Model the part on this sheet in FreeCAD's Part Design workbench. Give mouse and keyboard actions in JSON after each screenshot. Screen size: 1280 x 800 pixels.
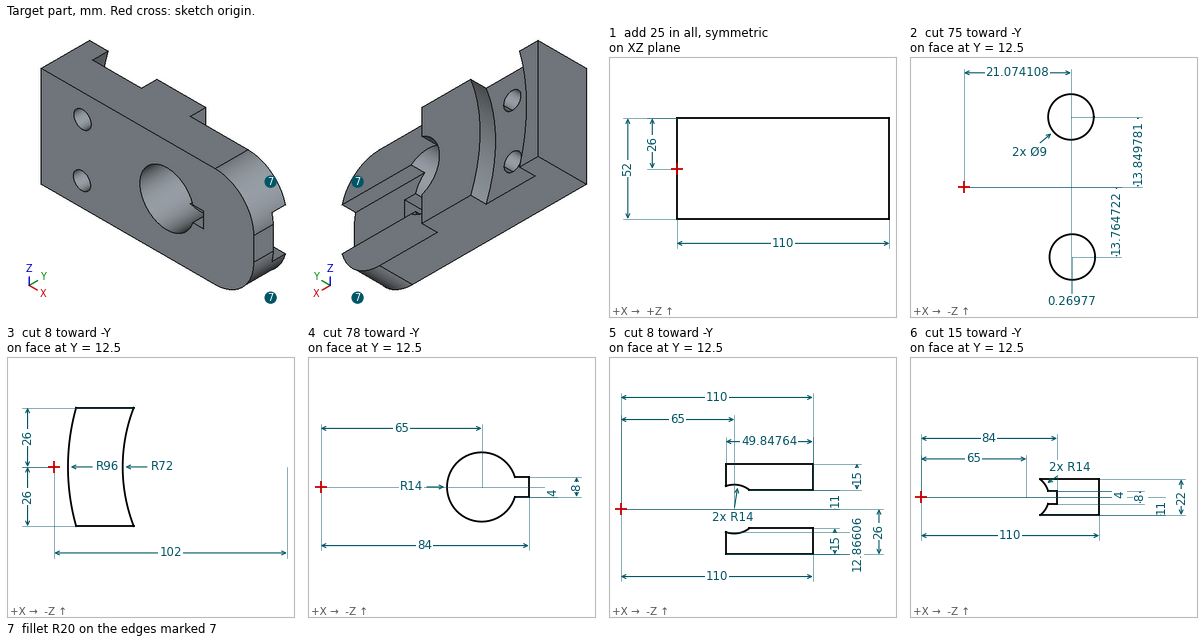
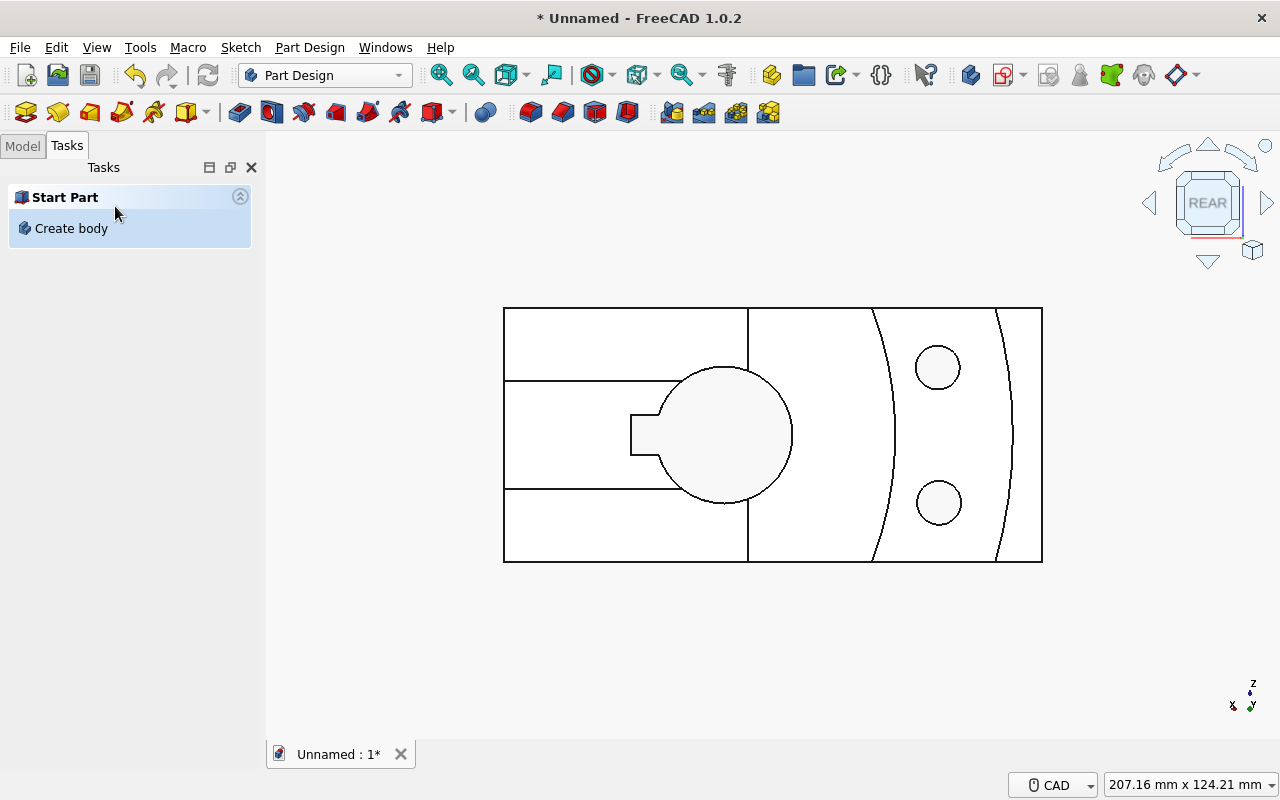
{"action": "left_click", "coordinate": [822, 507]}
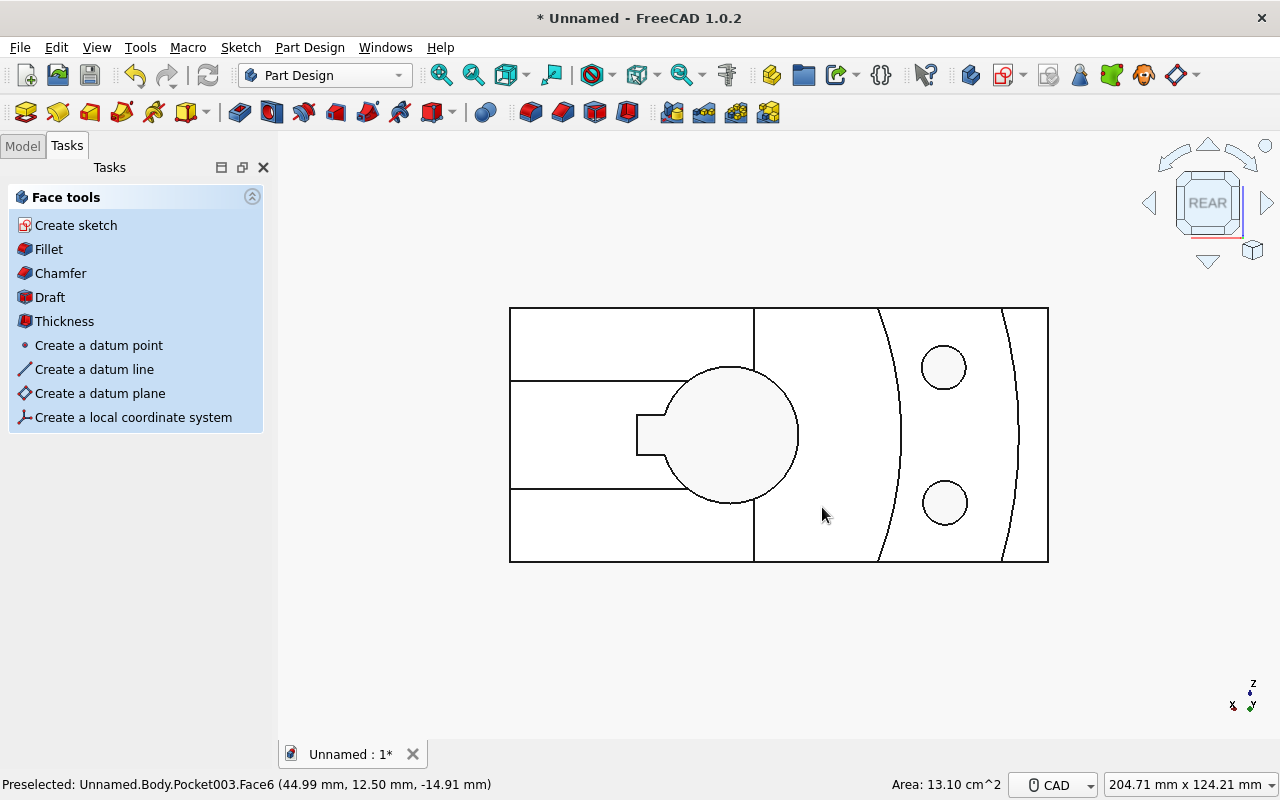
{"action": "left_click", "coordinate": [1004, 76]}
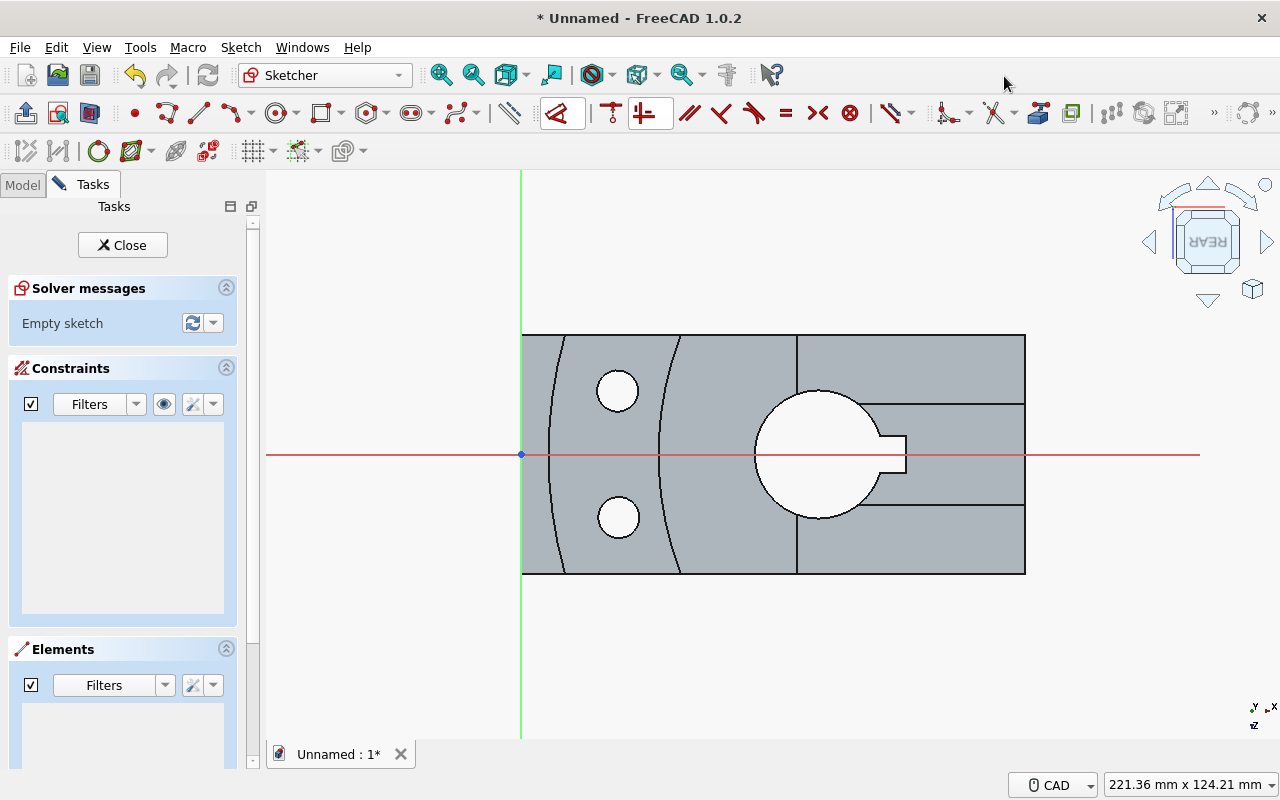
{"action": "scroll", "coordinate": [1044, 454], "scroll_direction": "up", "scroll_amount": 6}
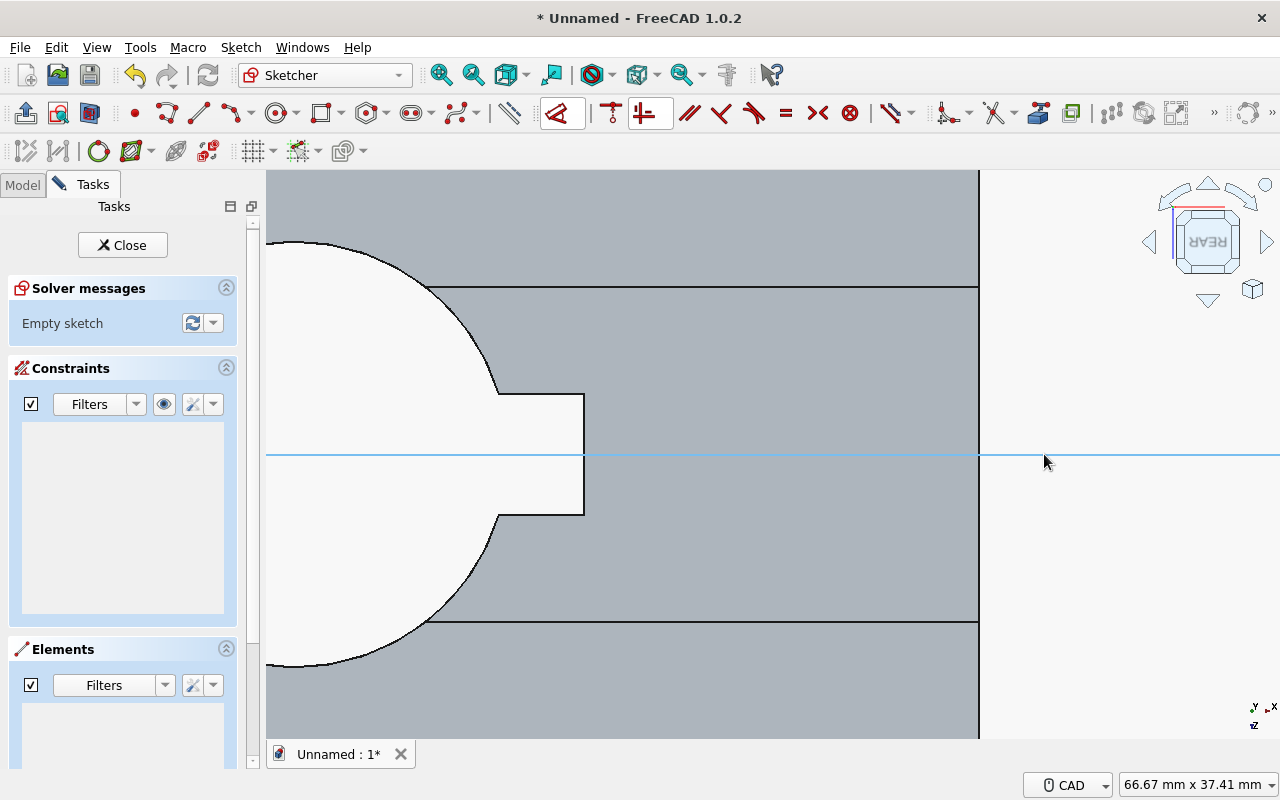
{"action": "left_click", "coordinate": [168, 114]}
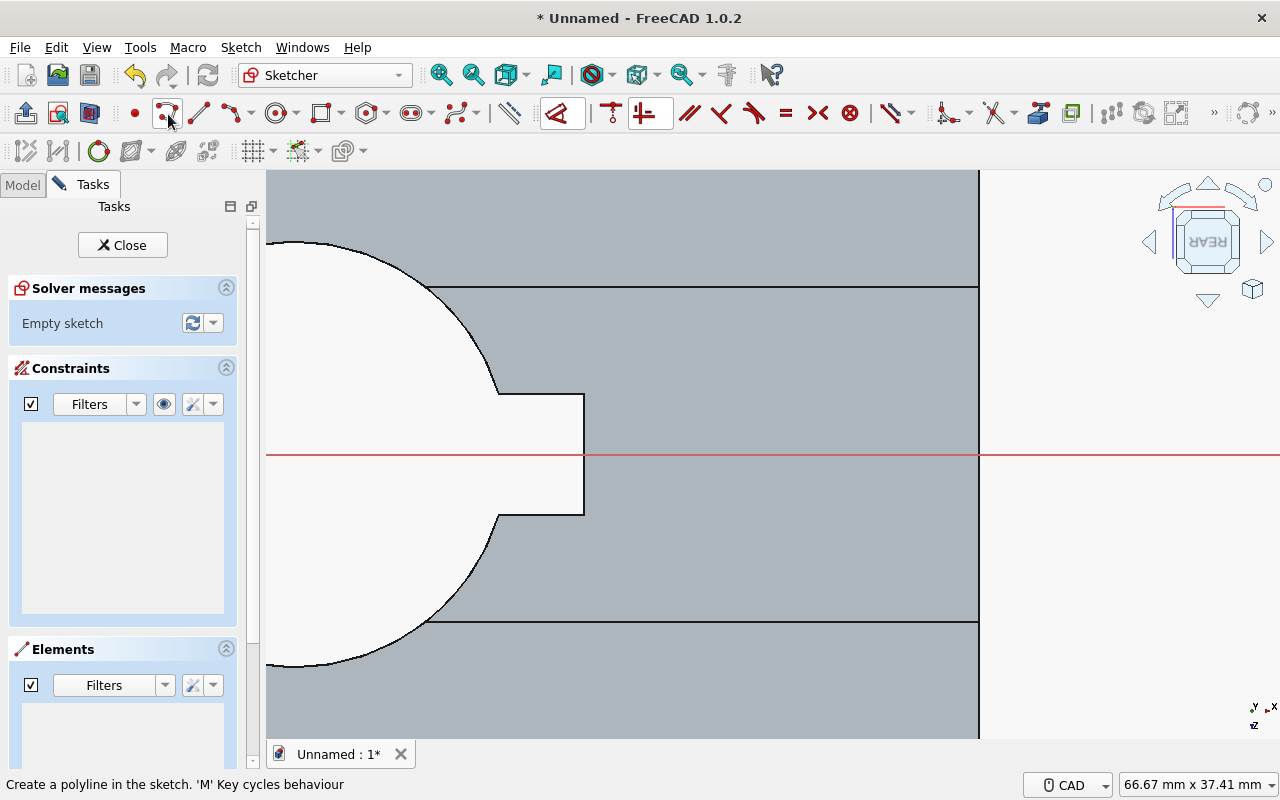
{"action": "left_click", "coordinate": [499, 394]}
{"action": "left_click", "coordinate": [584, 394]}
{"action": "left_click", "coordinate": [584, 515]}
{"action": "left_click", "coordinate": [499, 515]}
{"action": "right_click", "coordinate": [499, 515]}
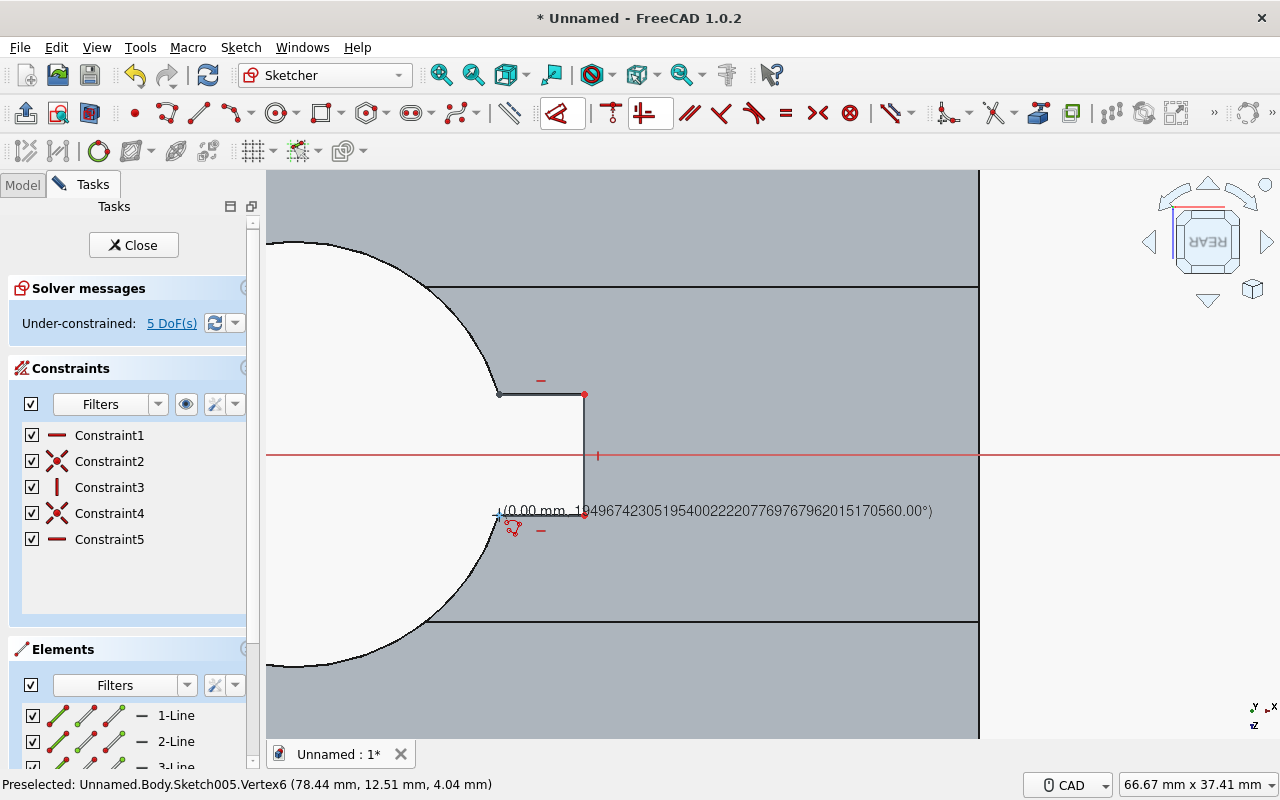
{"action": "left_click", "coordinate": [426, 622]}
{"action": "left_click", "coordinate": [979, 622]}
{"action": "left_click", "coordinate": [979, 287]}
{"action": "left_click", "coordinate": [426, 287]}
{"action": "right_click", "coordinate": [426, 287]}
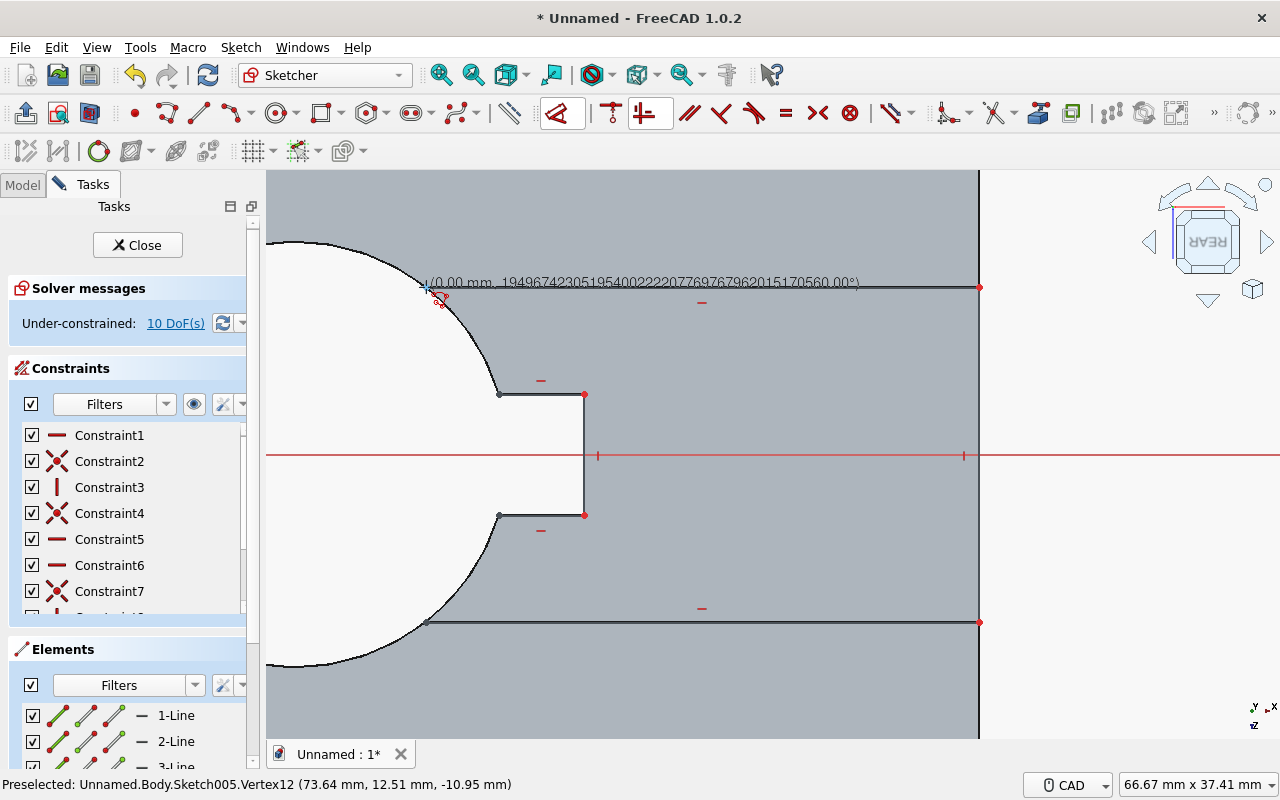
{"action": "left_click", "coordinate": [232, 114]}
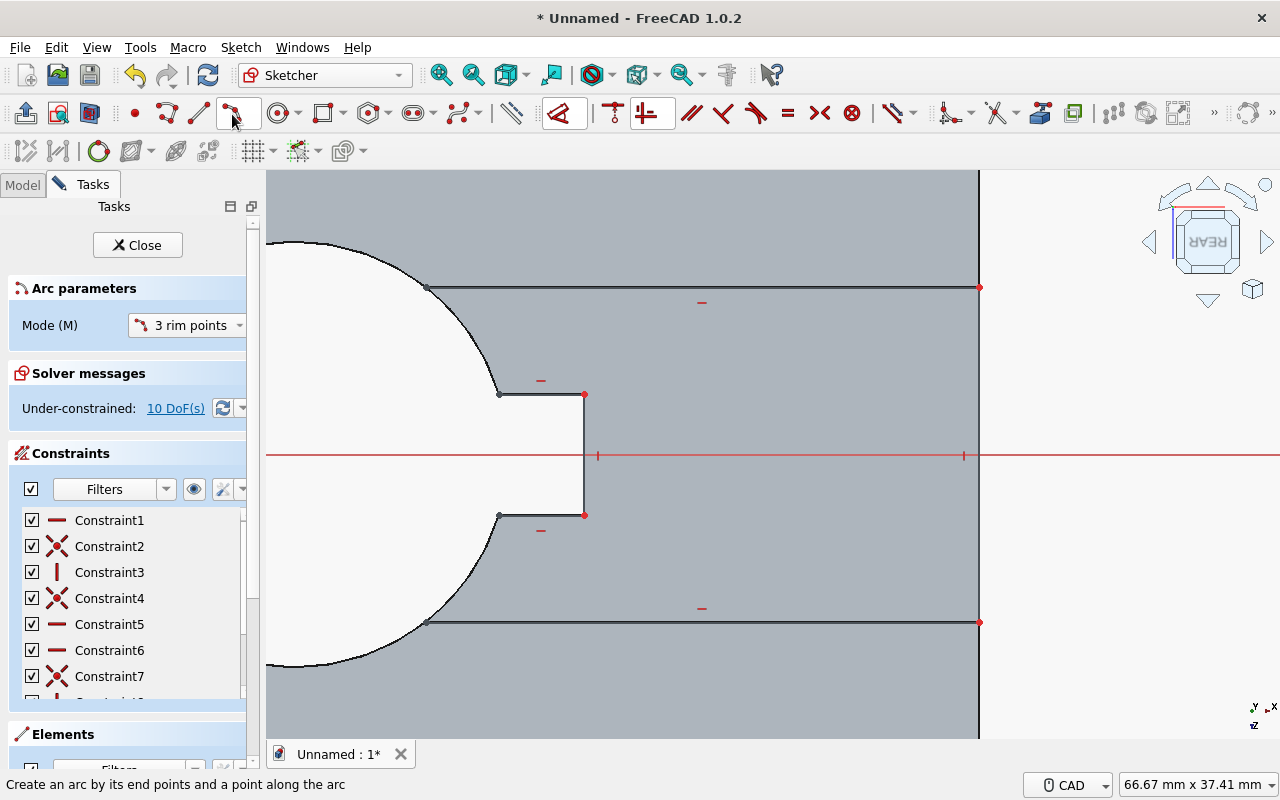
{"action": "left_click", "coordinate": [499, 516]}
{"action": "left_click", "coordinate": [426, 623]}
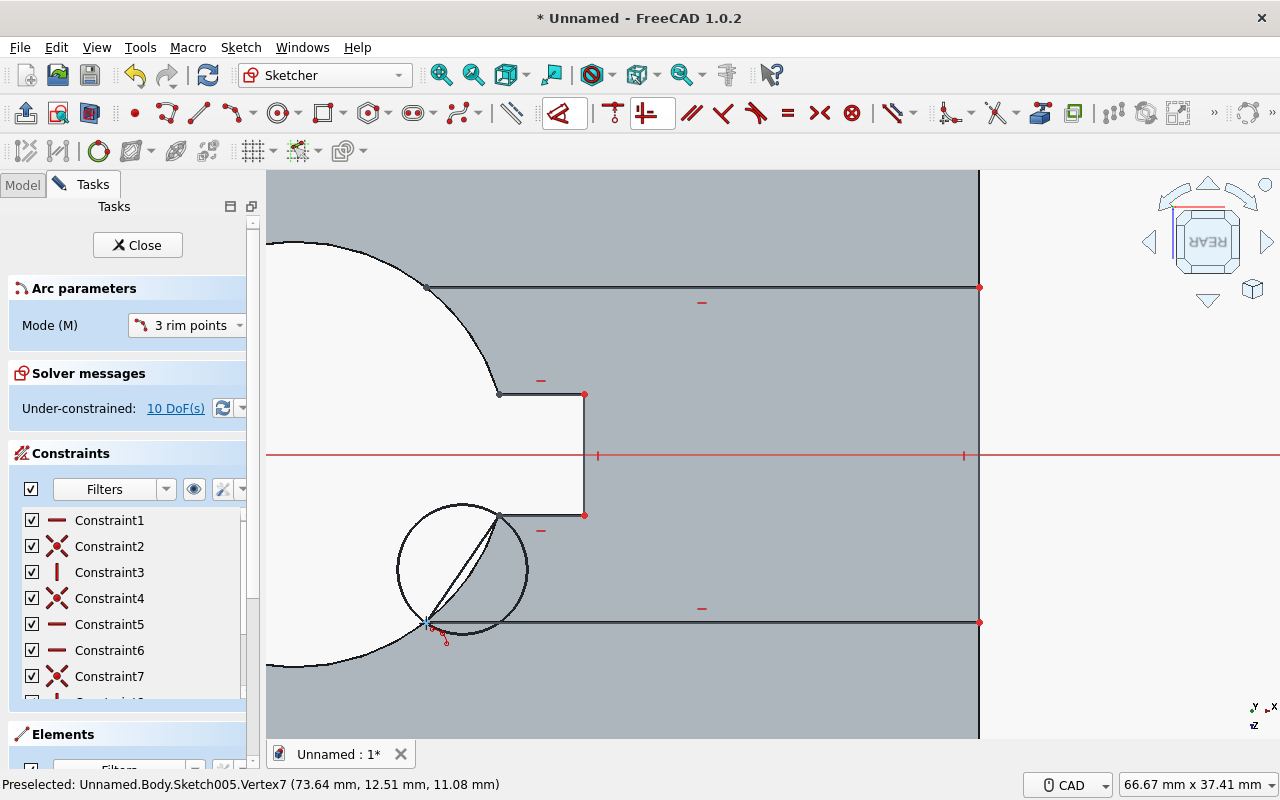
{"action": "scroll", "coordinate": [471, 574], "scroll_direction": "up", "scroll_amount": 3}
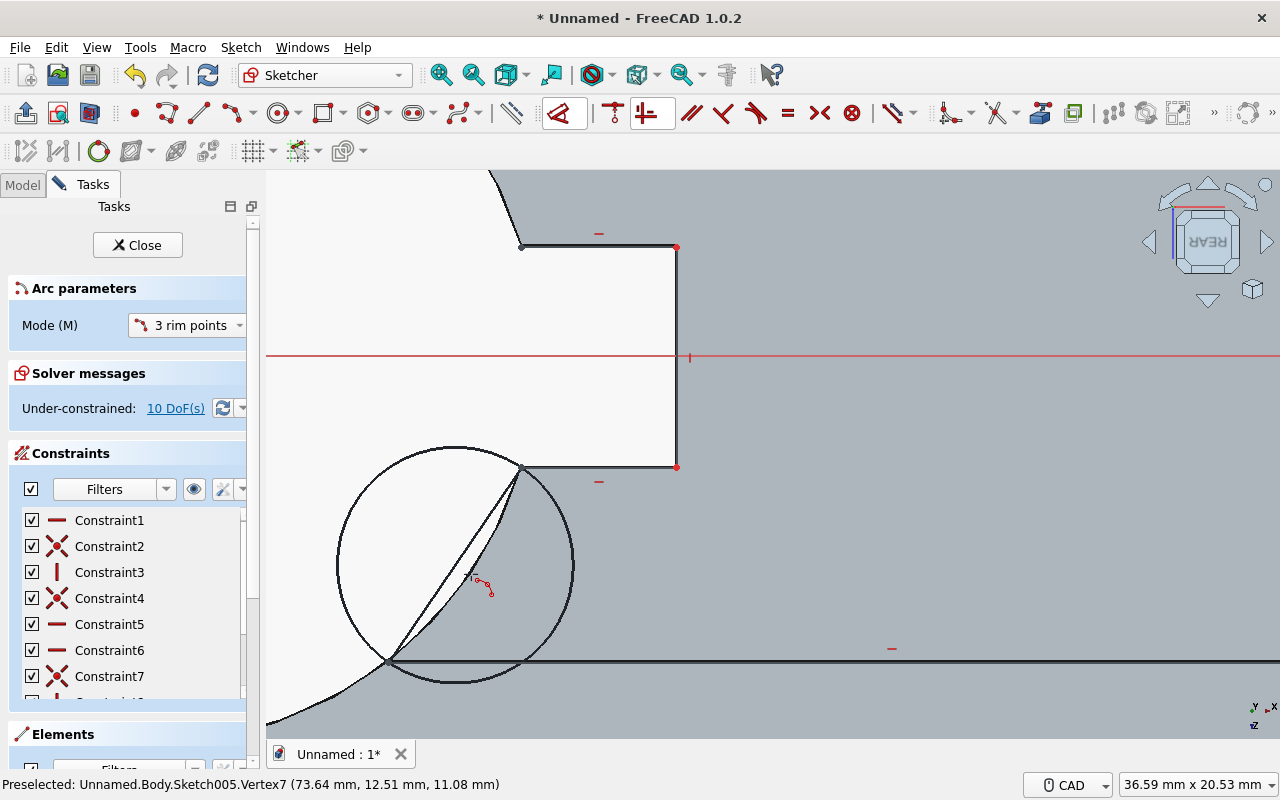
{"action": "left_click", "coordinate": [470, 574]}